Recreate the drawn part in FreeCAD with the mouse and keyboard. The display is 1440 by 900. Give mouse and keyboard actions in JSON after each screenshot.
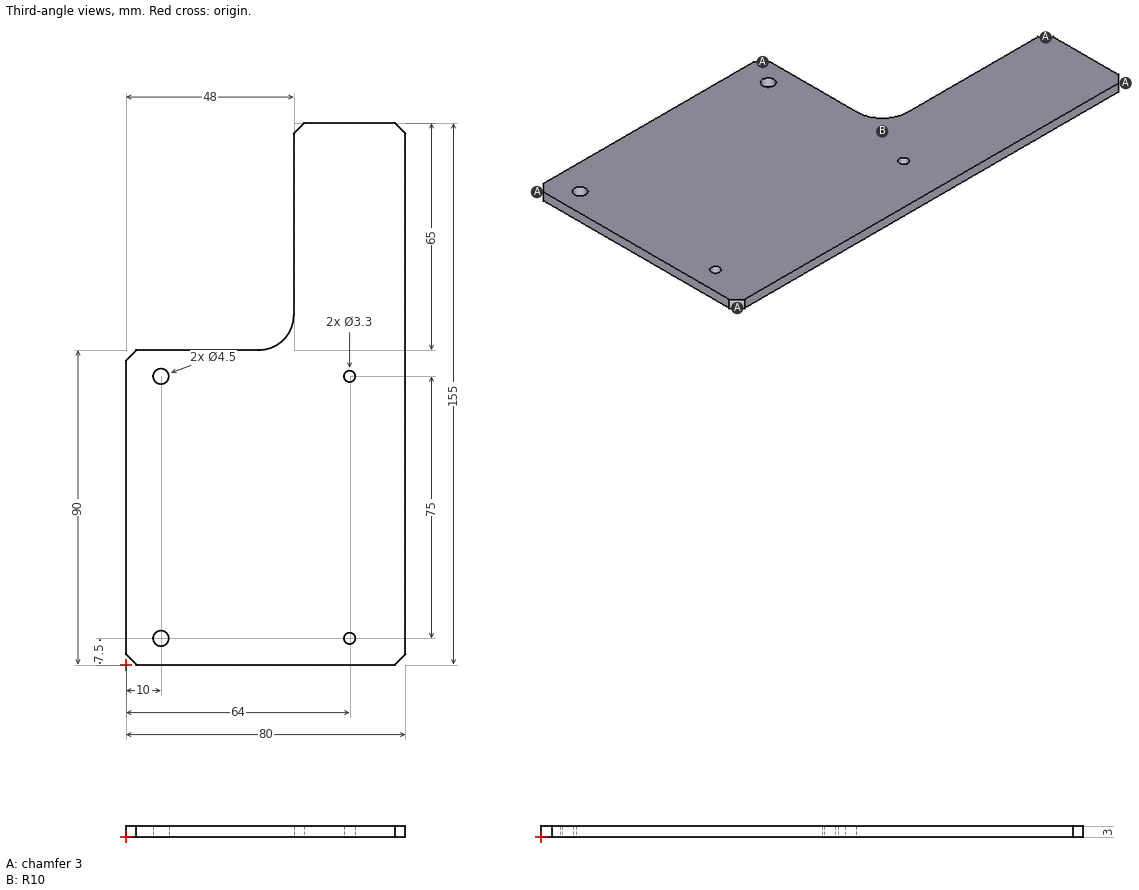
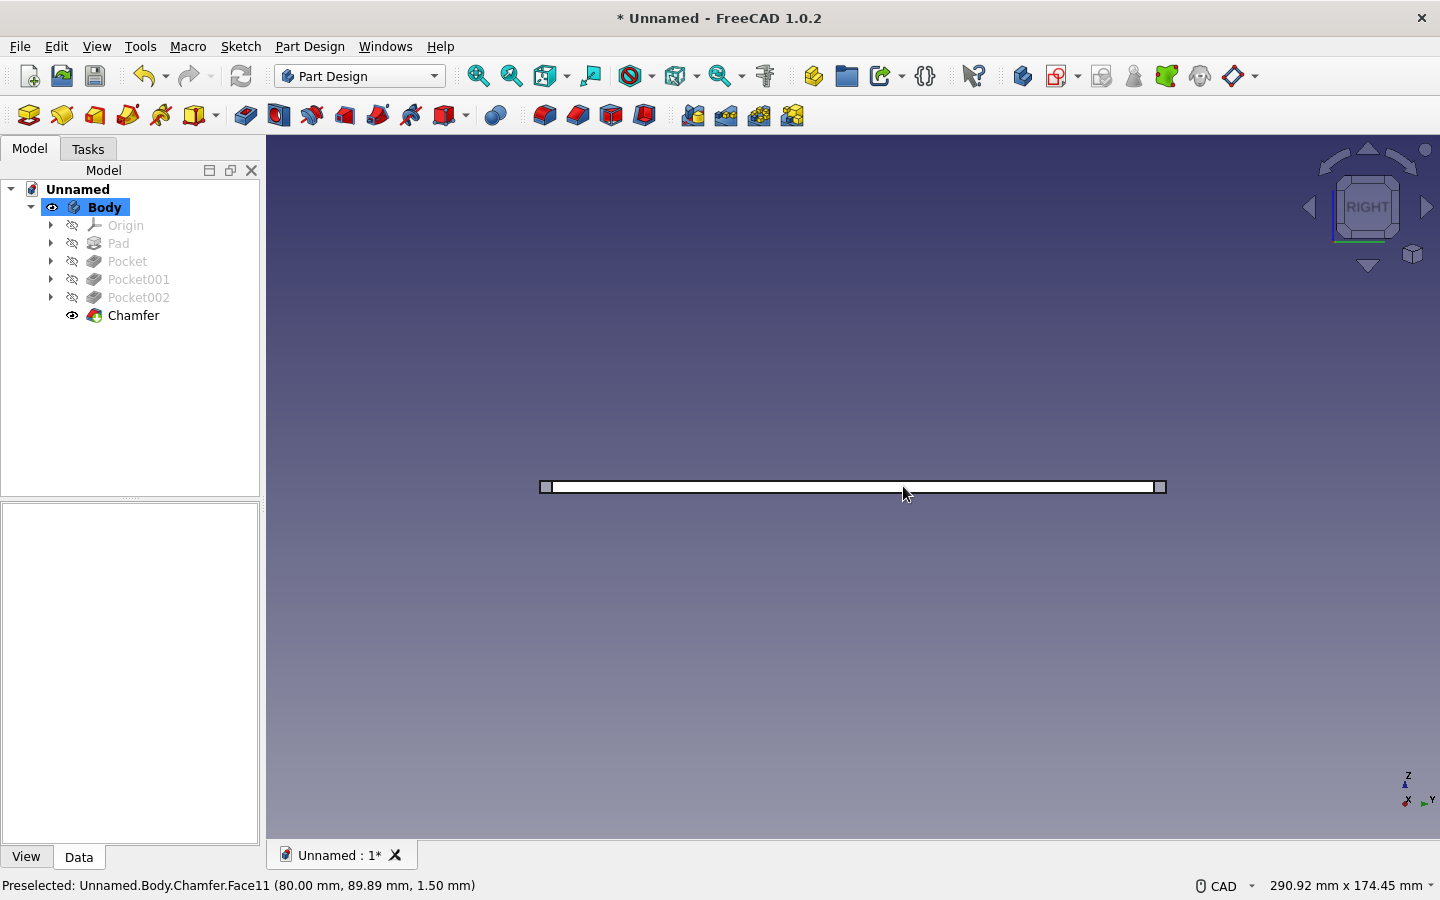
{"action": "key", "text": "5"}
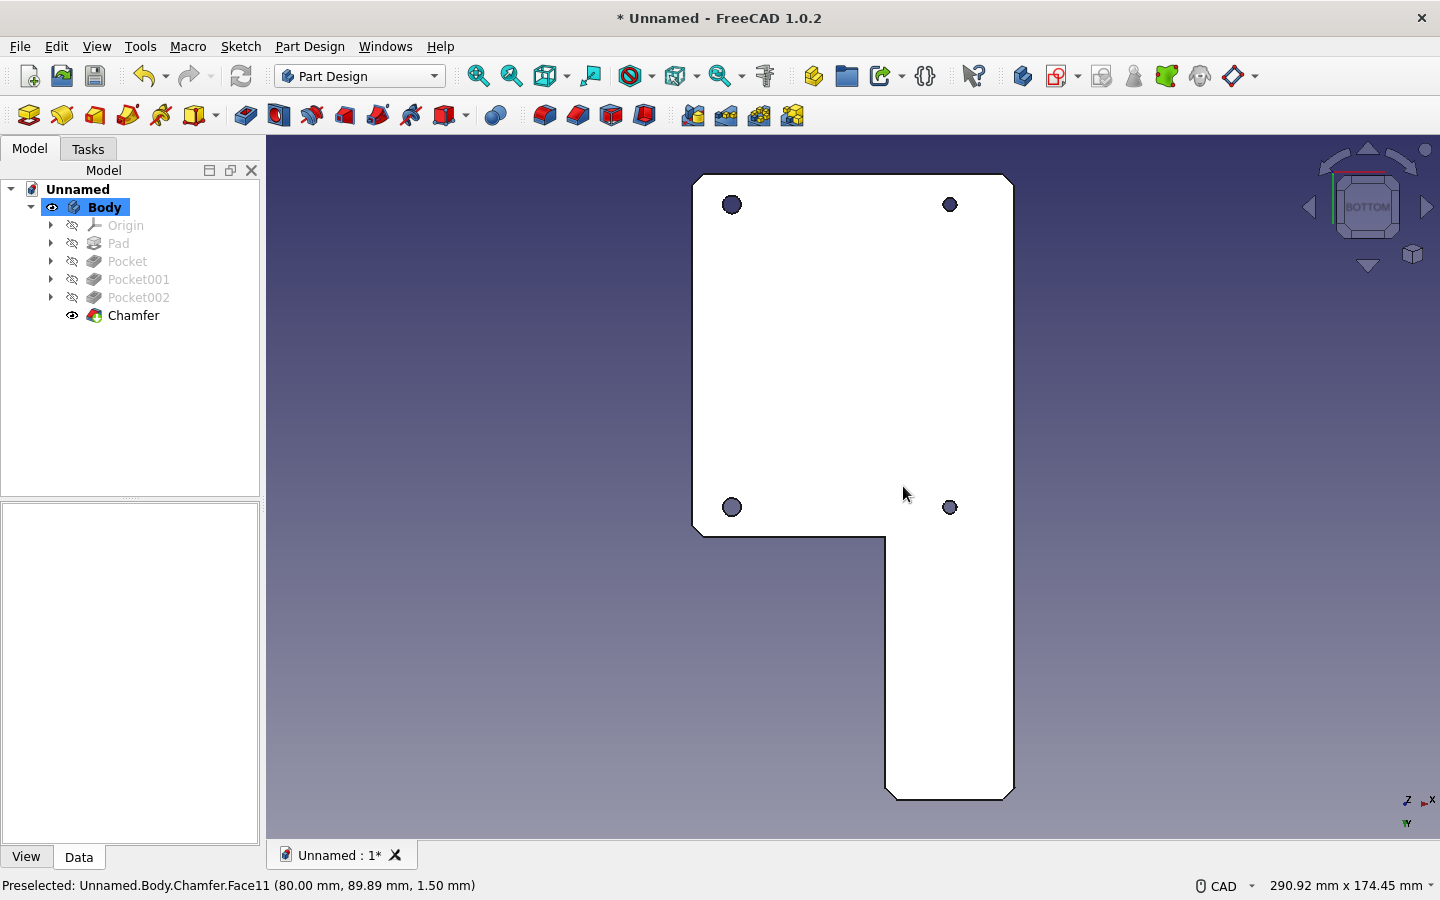
{"action": "scroll", "coordinate": [885, 536], "scroll_direction": "up", "scroll_amount": 6}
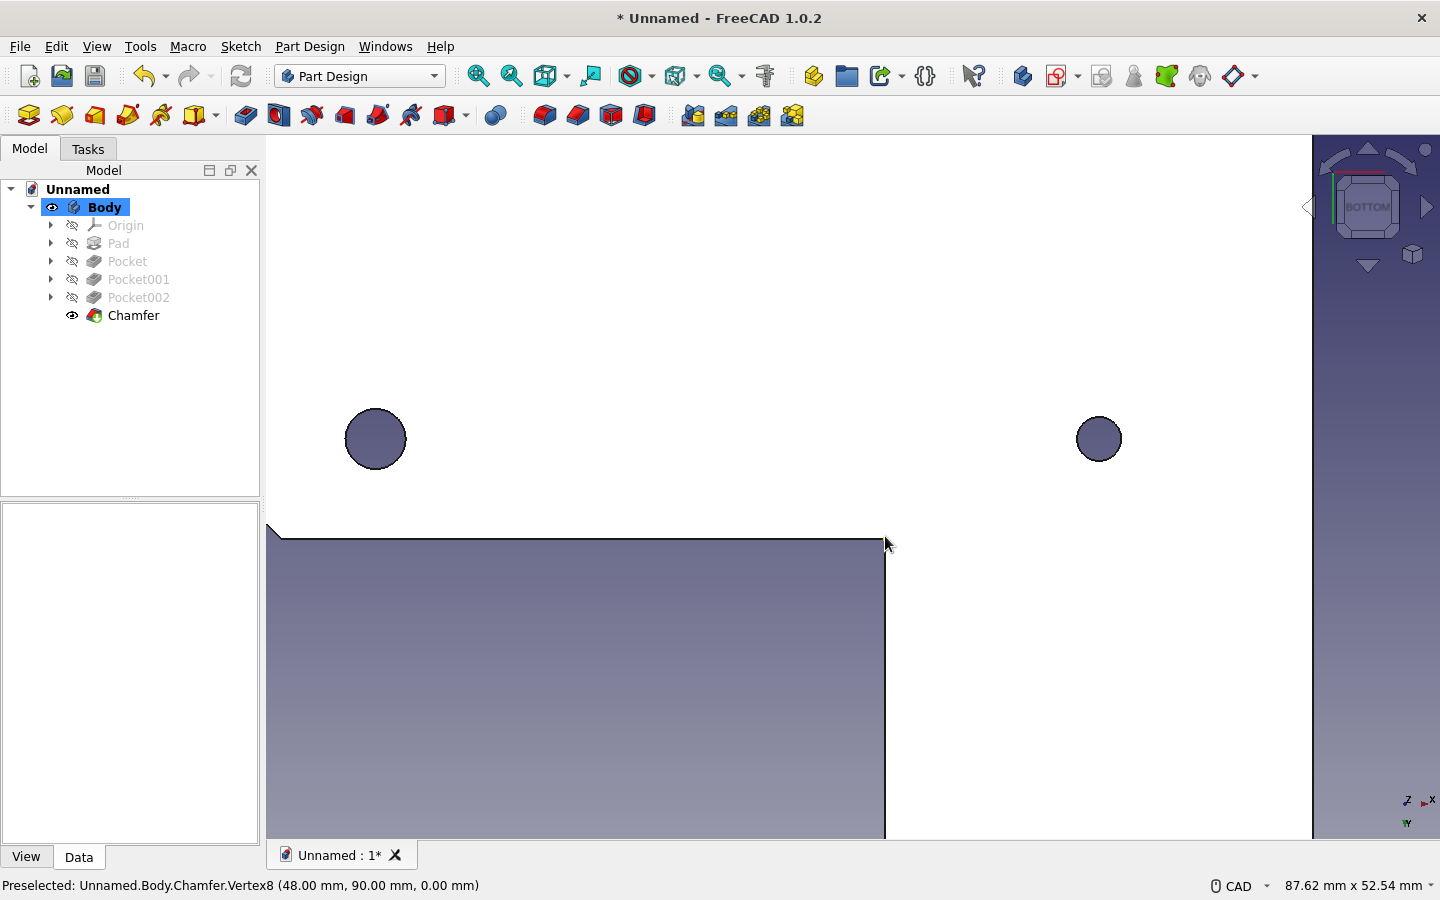
{"action": "key", "text": "v f"}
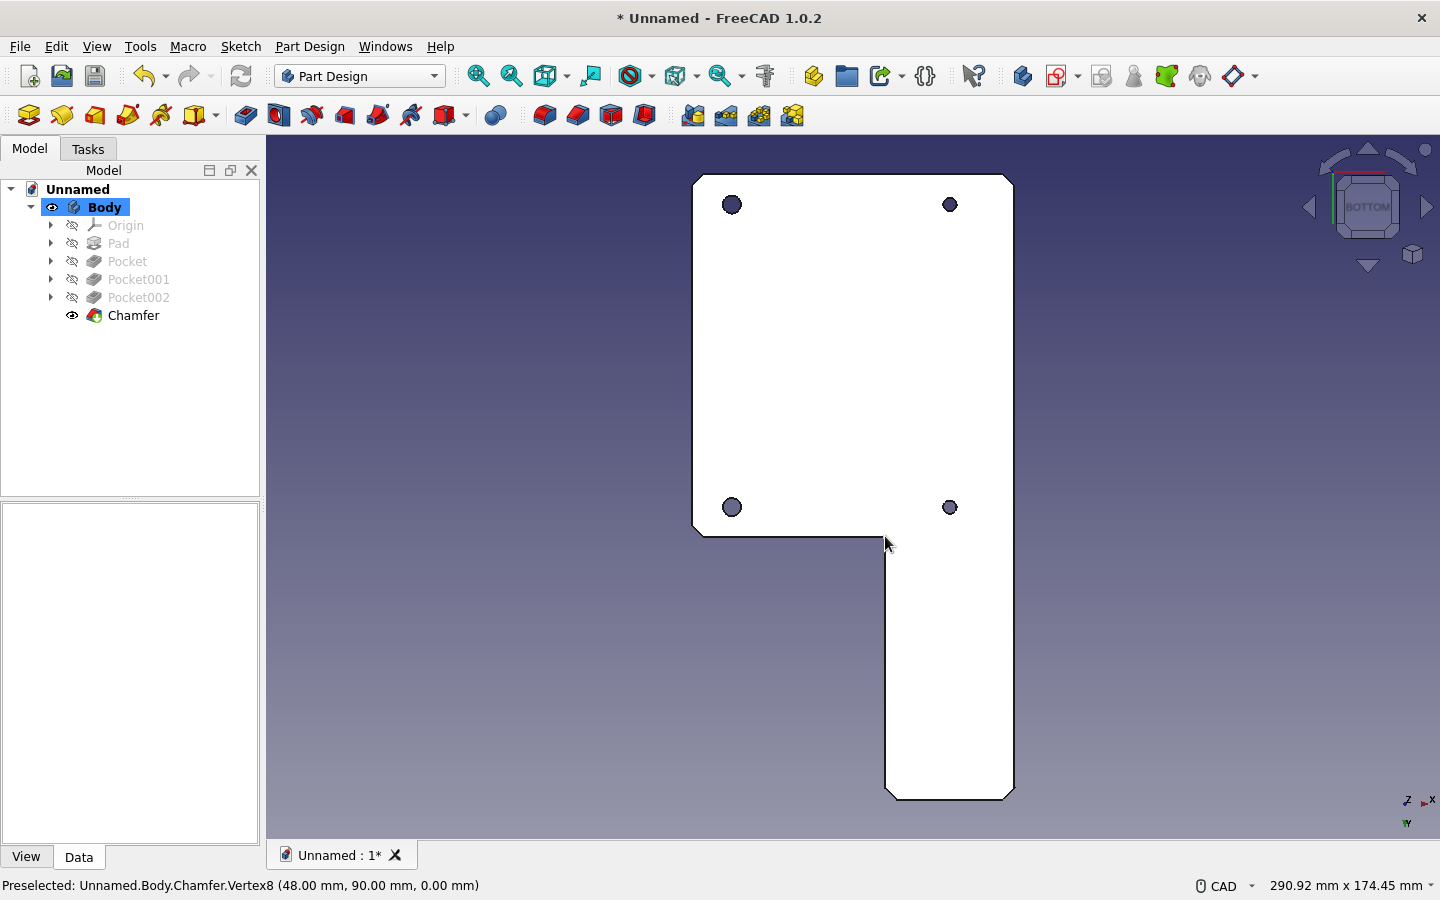
{"action": "key", "text": "4"}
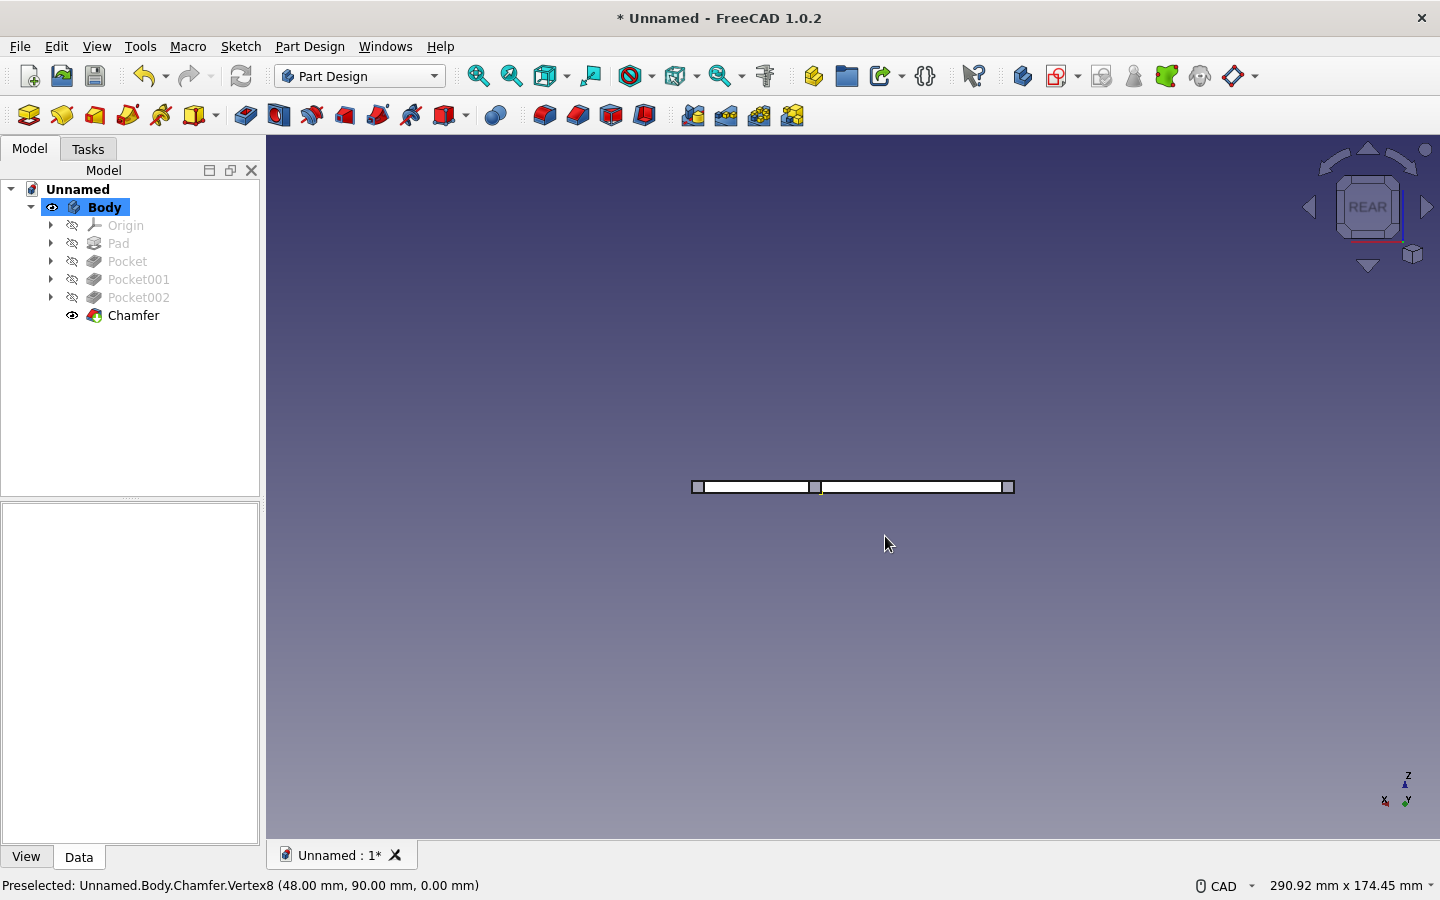
{"action": "key", "text": "v f"}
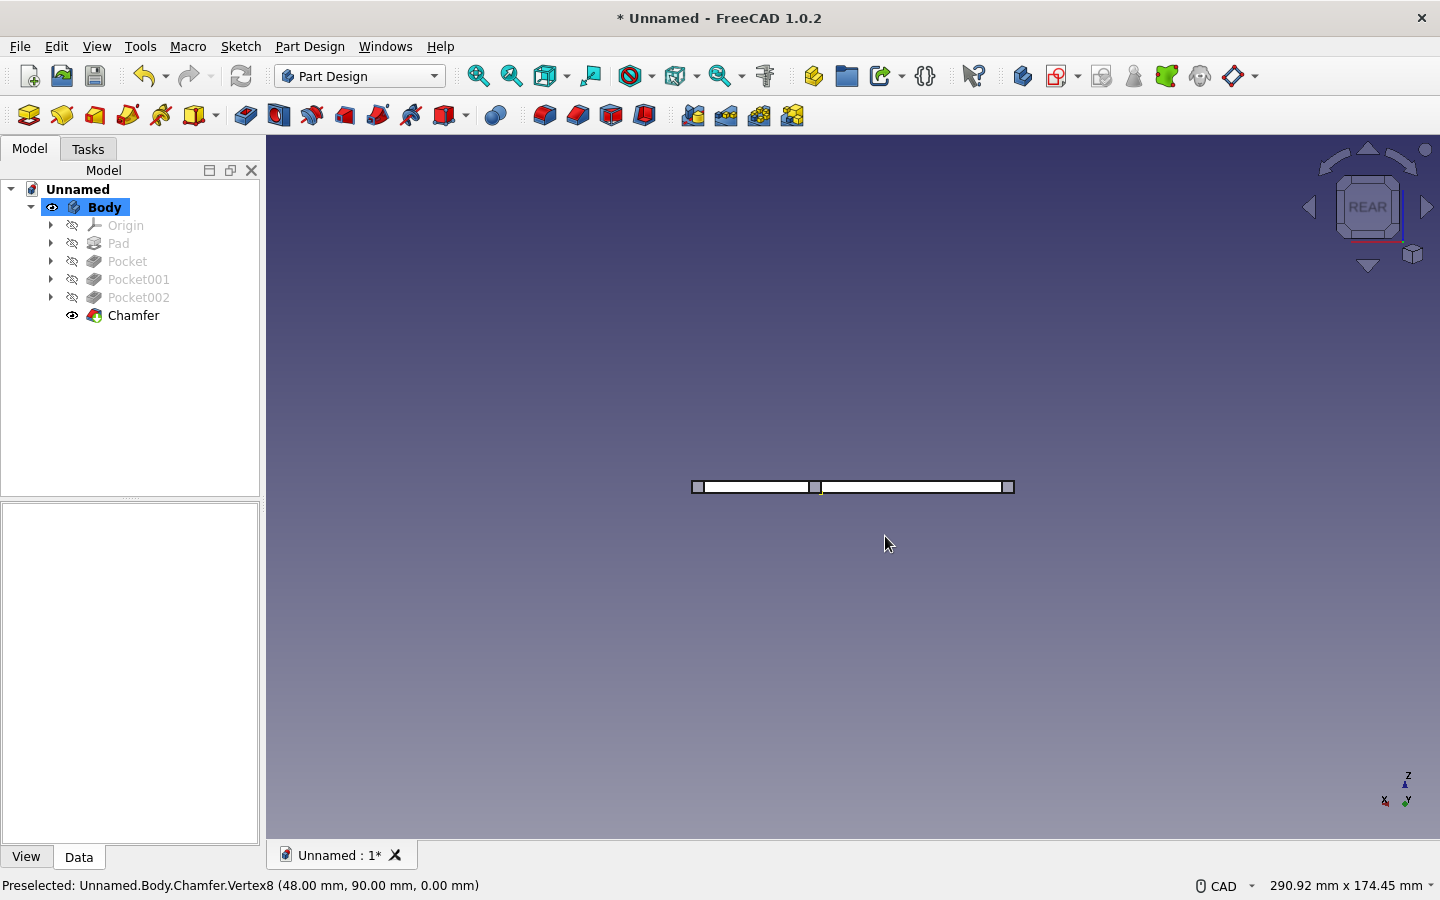
{"action": "scroll", "coordinate": [821, 486], "scroll_direction": "up", "scroll_amount": 6}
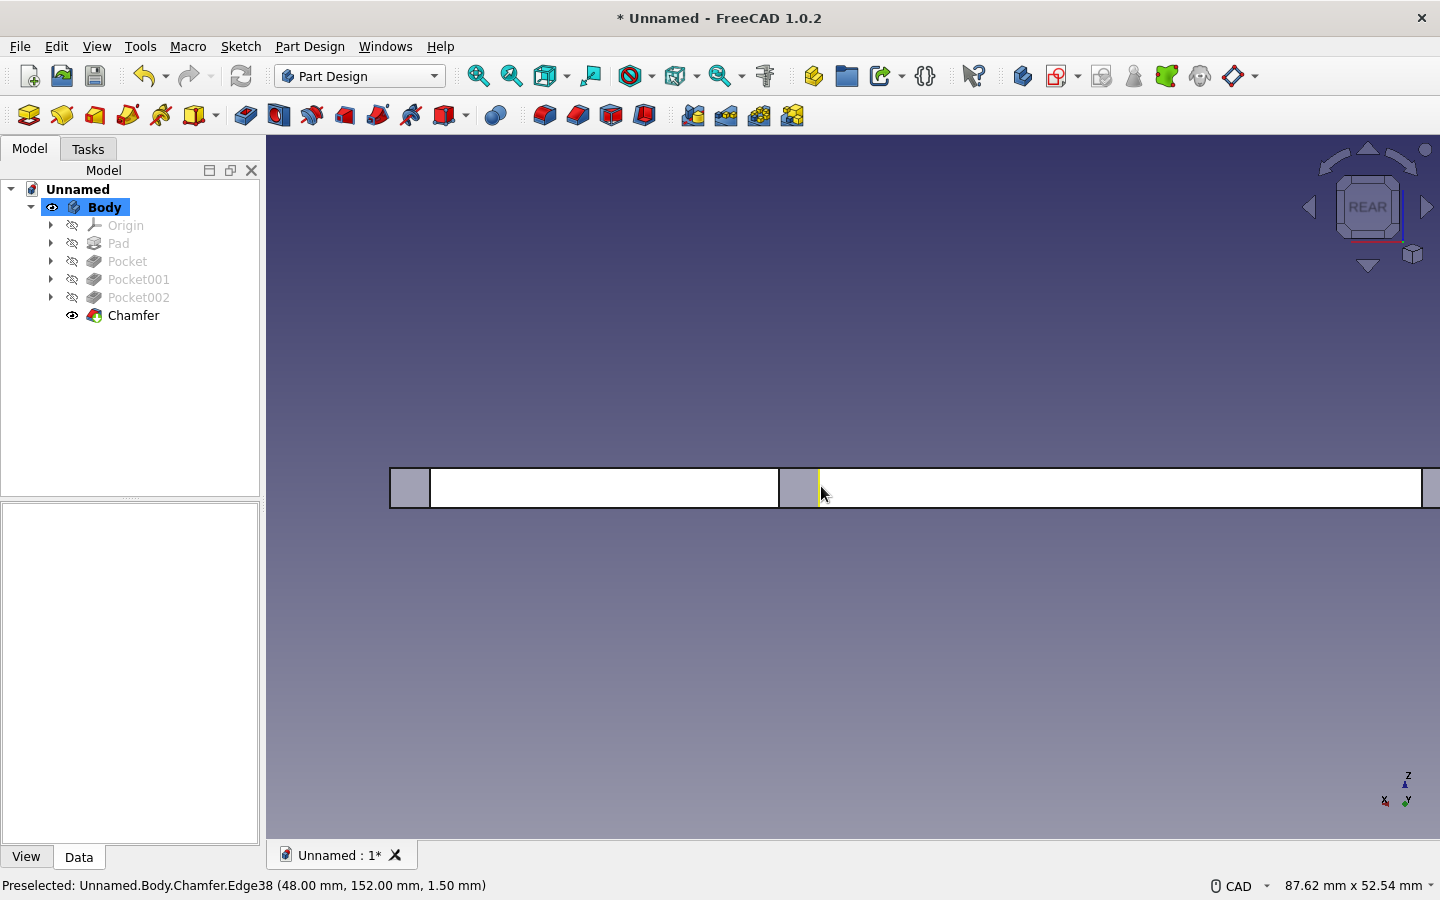
{"action": "key", "text": "v f"}